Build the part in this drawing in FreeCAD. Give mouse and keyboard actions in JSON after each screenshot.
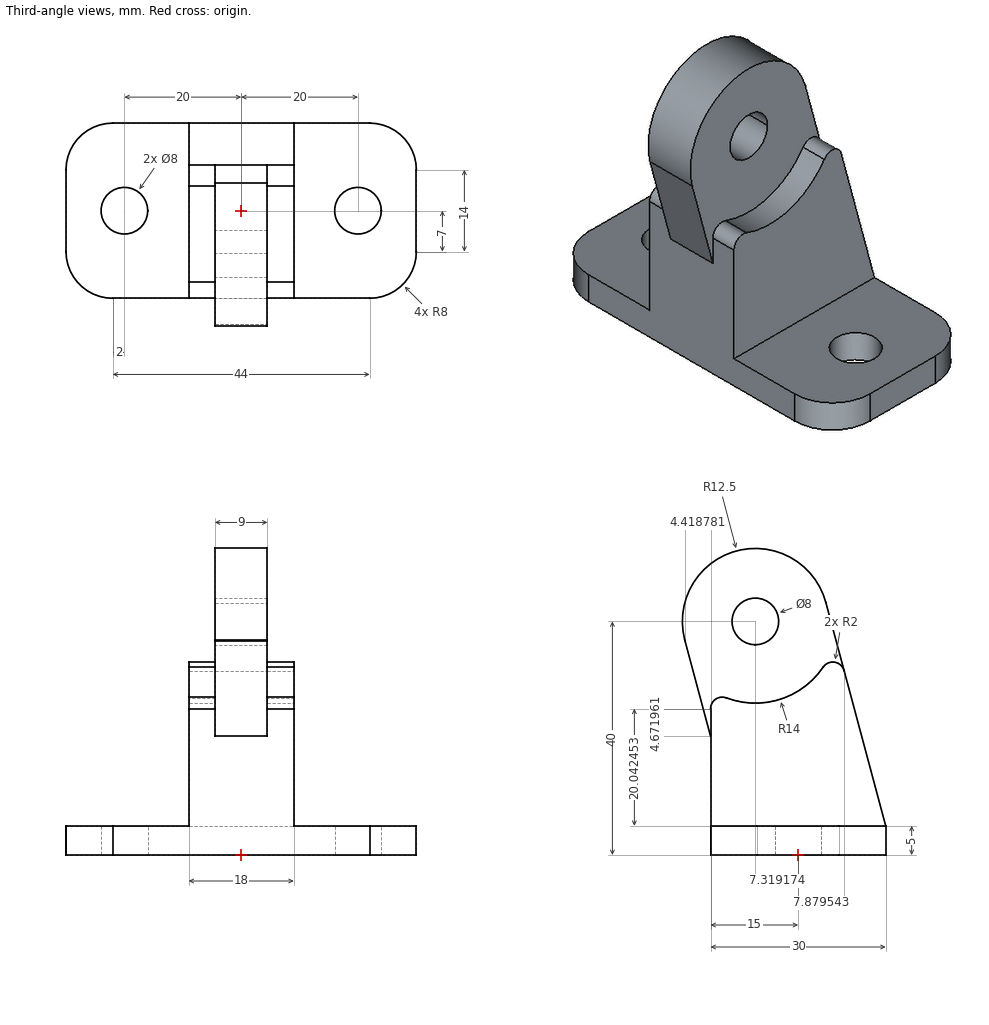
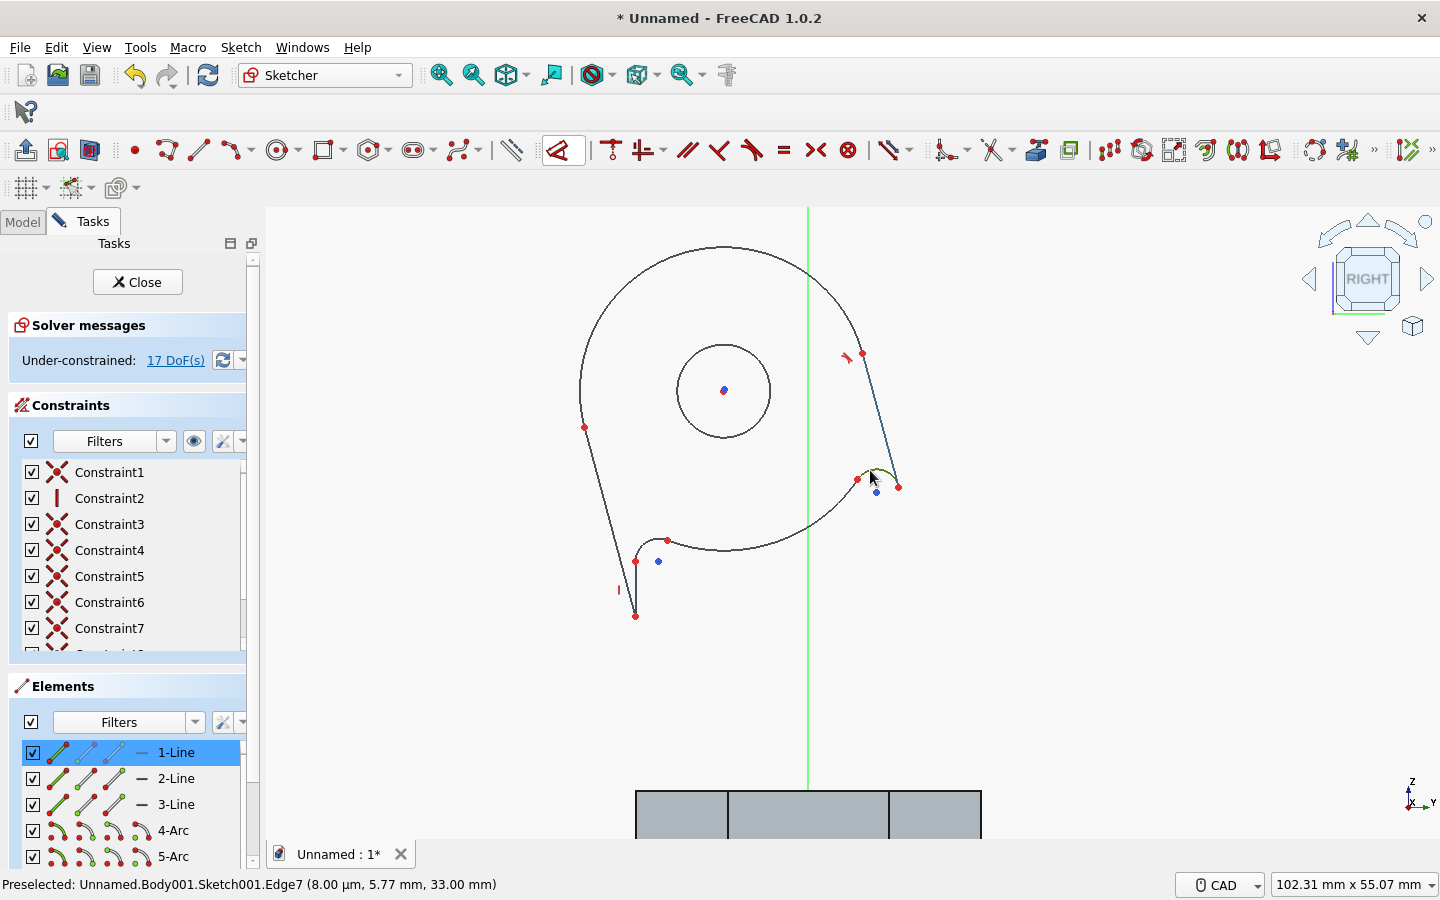
{"action": "left_click", "coordinate": [752, 150]}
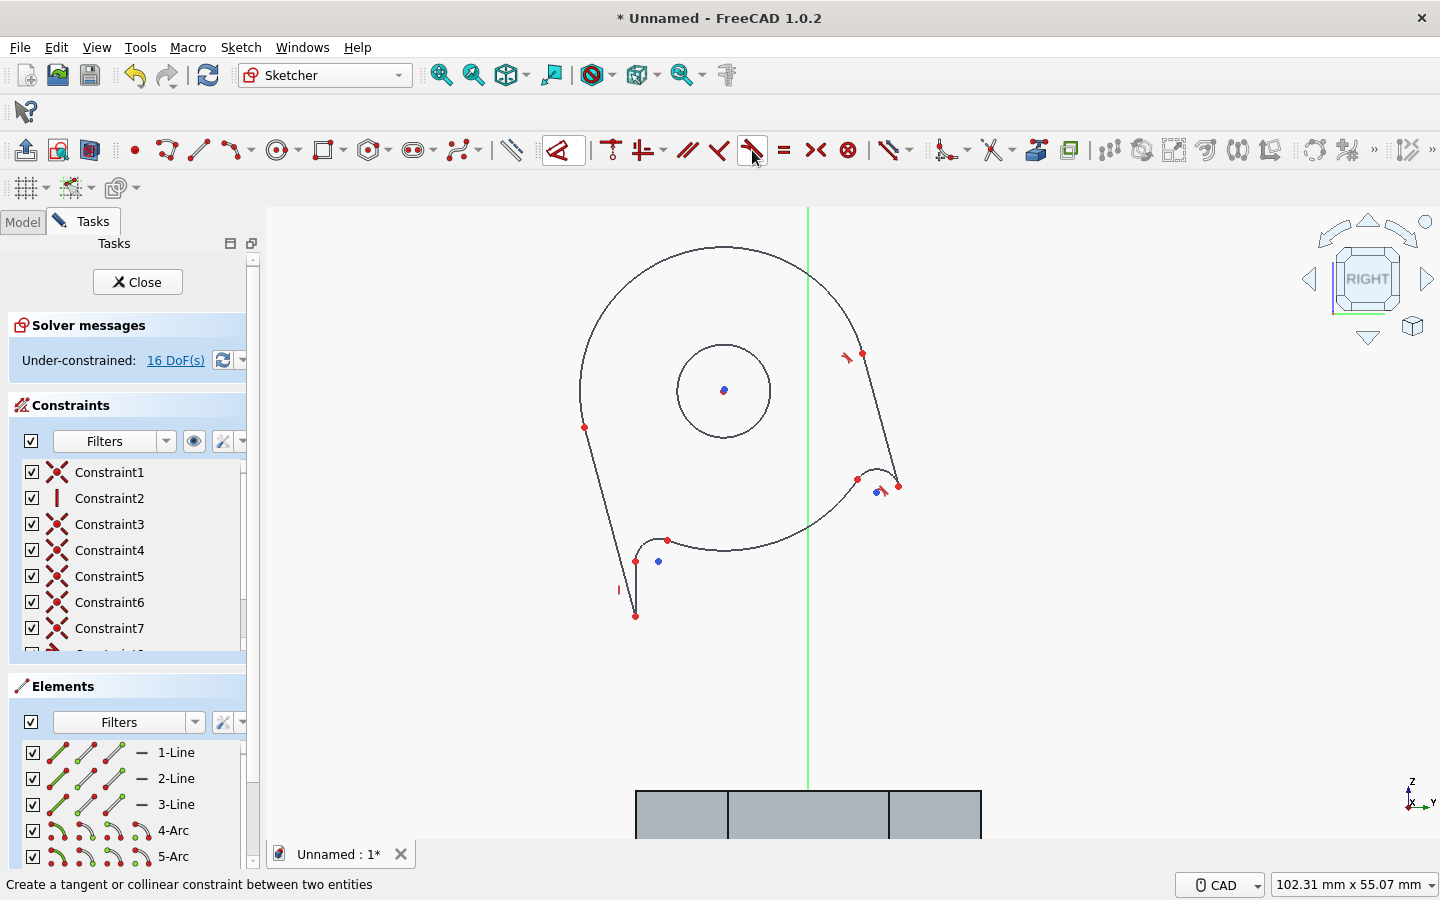
{"action": "scroll", "coordinate": [636, 578], "scroll_direction": "up", "scroll_amount": 2}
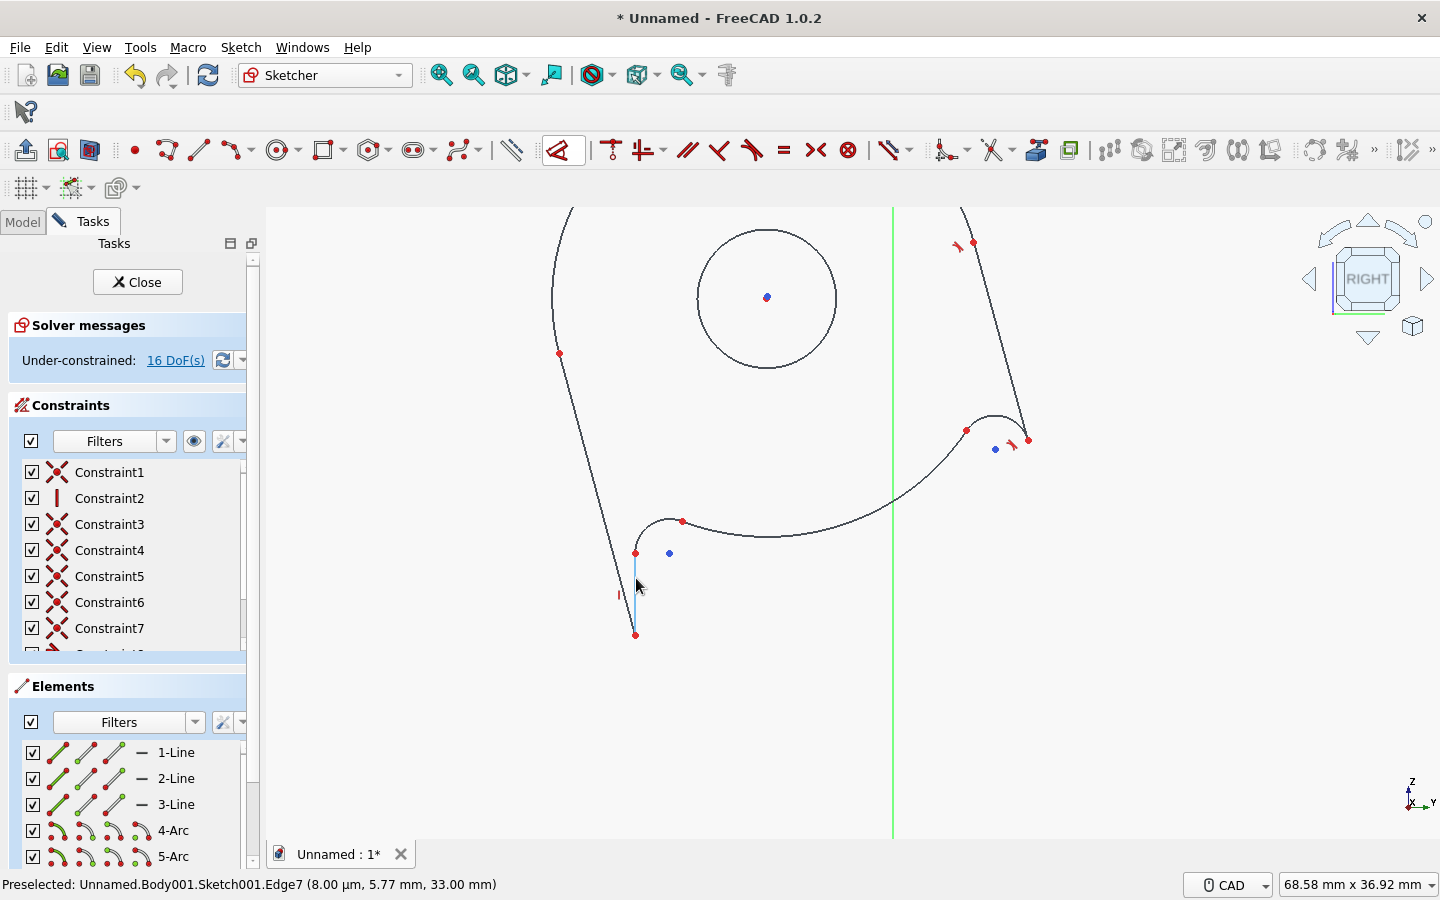
{"action": "left_click", "coordinate": [635, 578]}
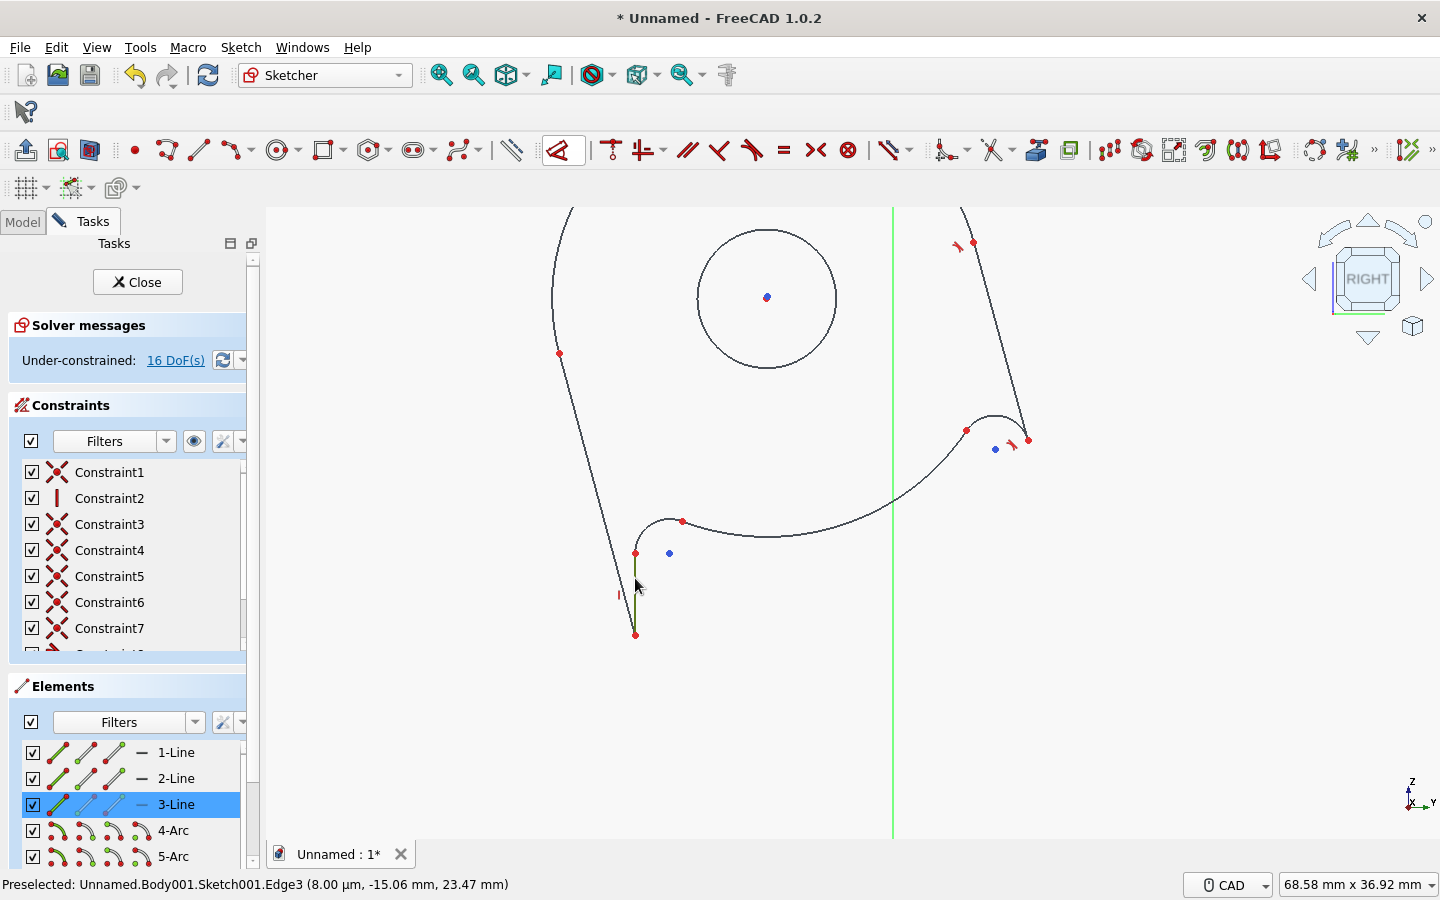
{"action": "left_click", "coordinate": [663, 520]}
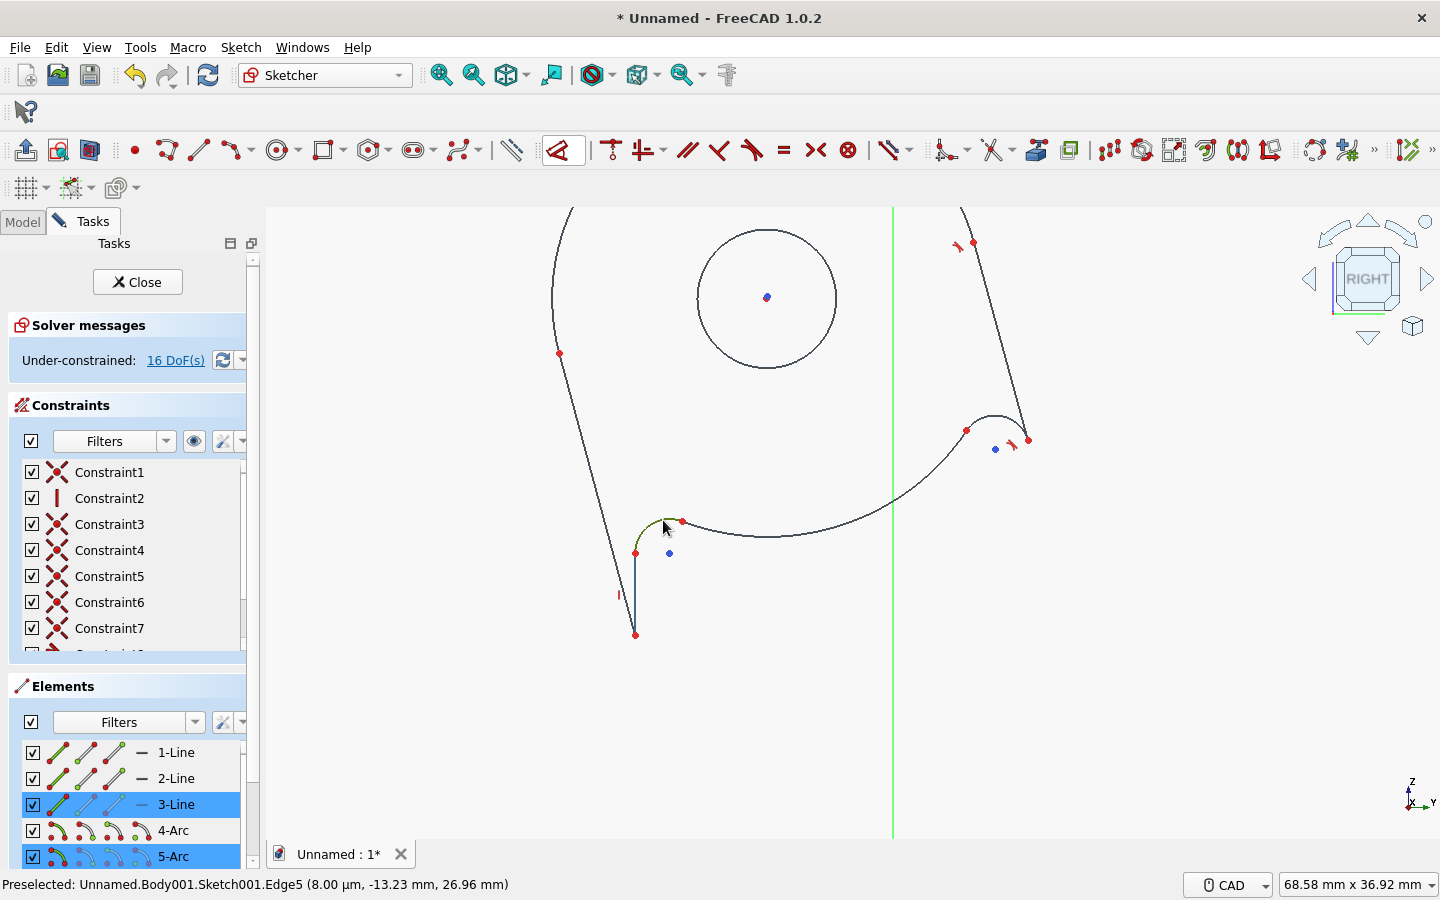
{"action": "key", "text": "t"}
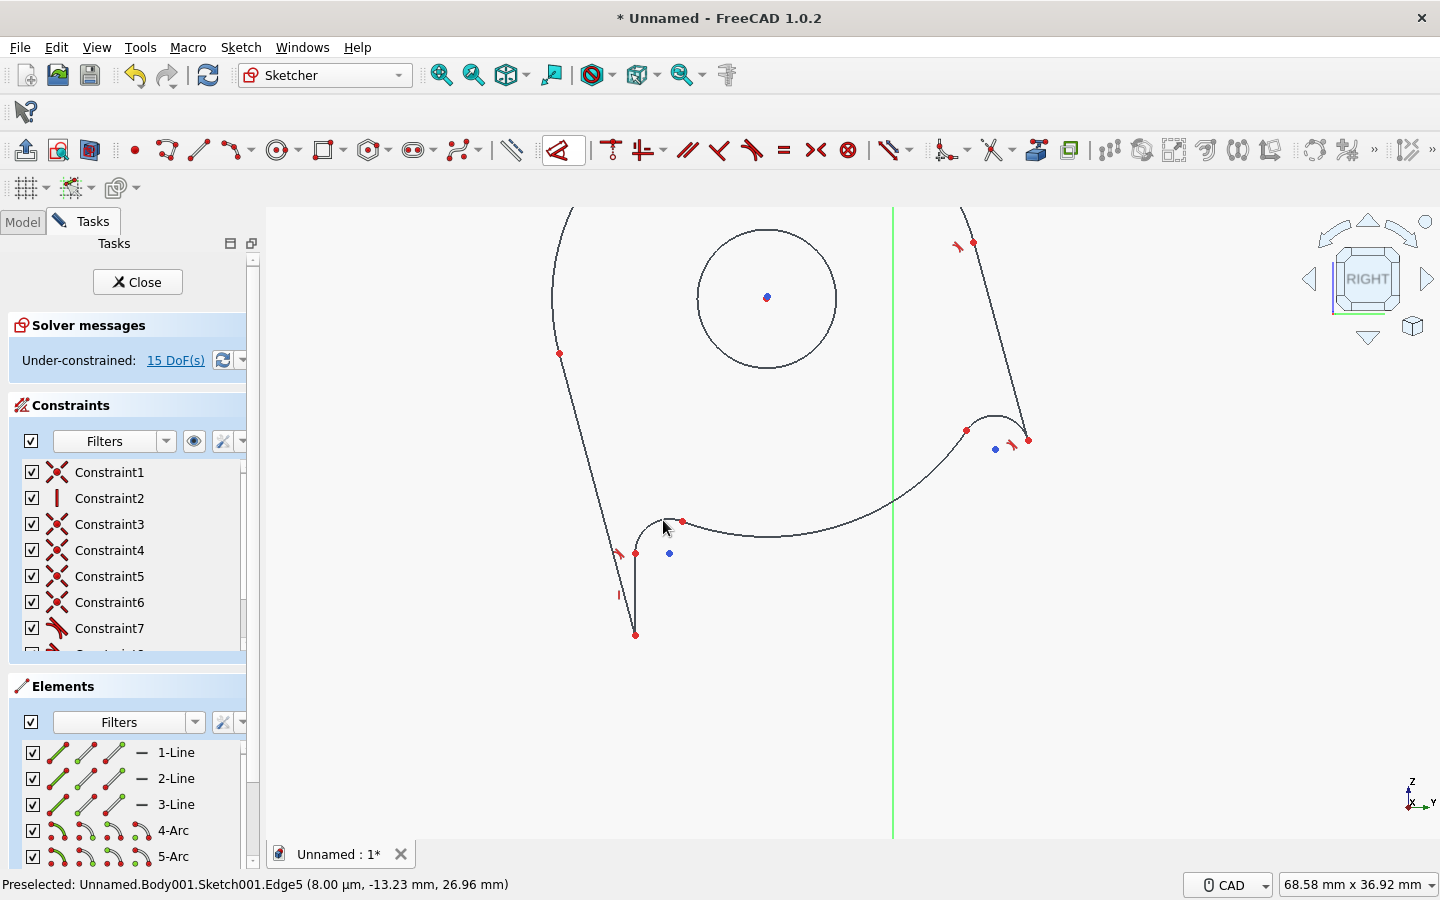
{"action": "left_click", "coordinate": [662, 520]}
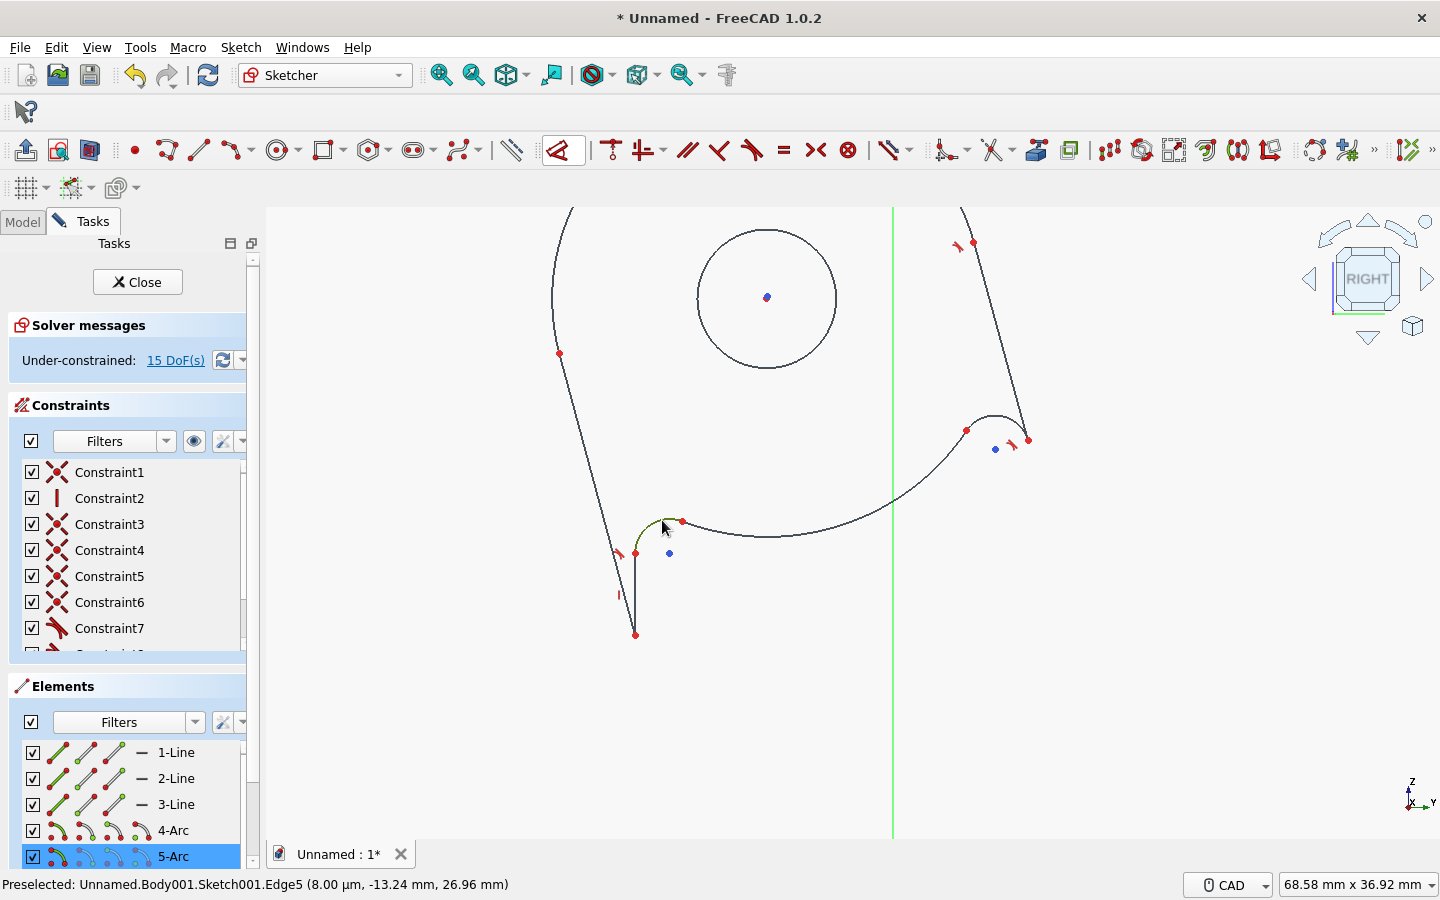
{"action": "left_click", "coordinate": [777, 537]}